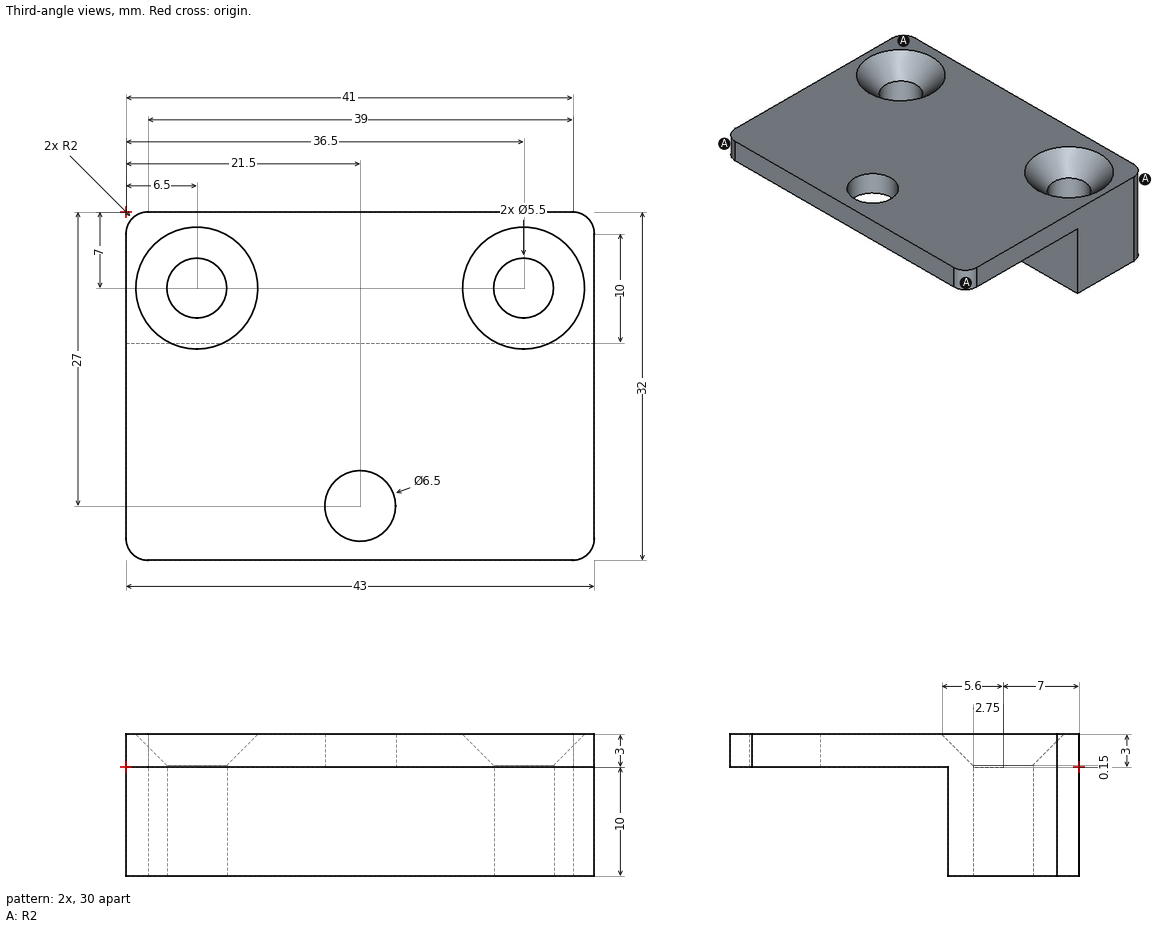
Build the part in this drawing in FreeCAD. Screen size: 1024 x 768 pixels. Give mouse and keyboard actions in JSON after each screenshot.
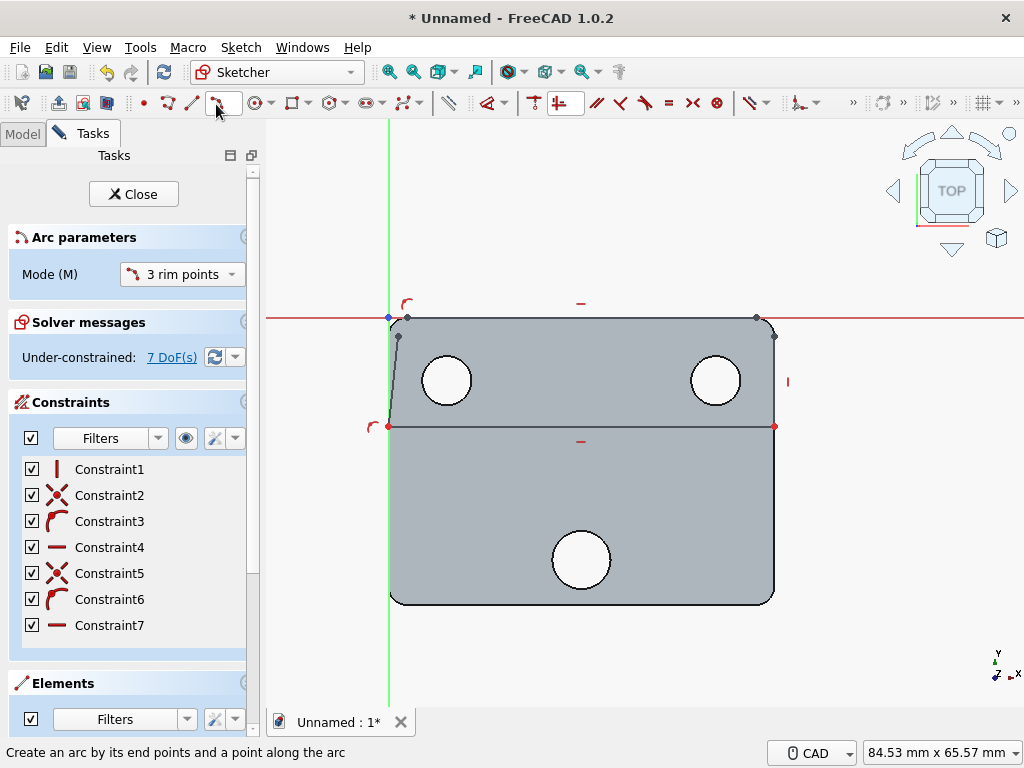
{"action": "left_click", "coordinate": [398, 337]}
{"action": "left_click", "coordinate": [407, 318]}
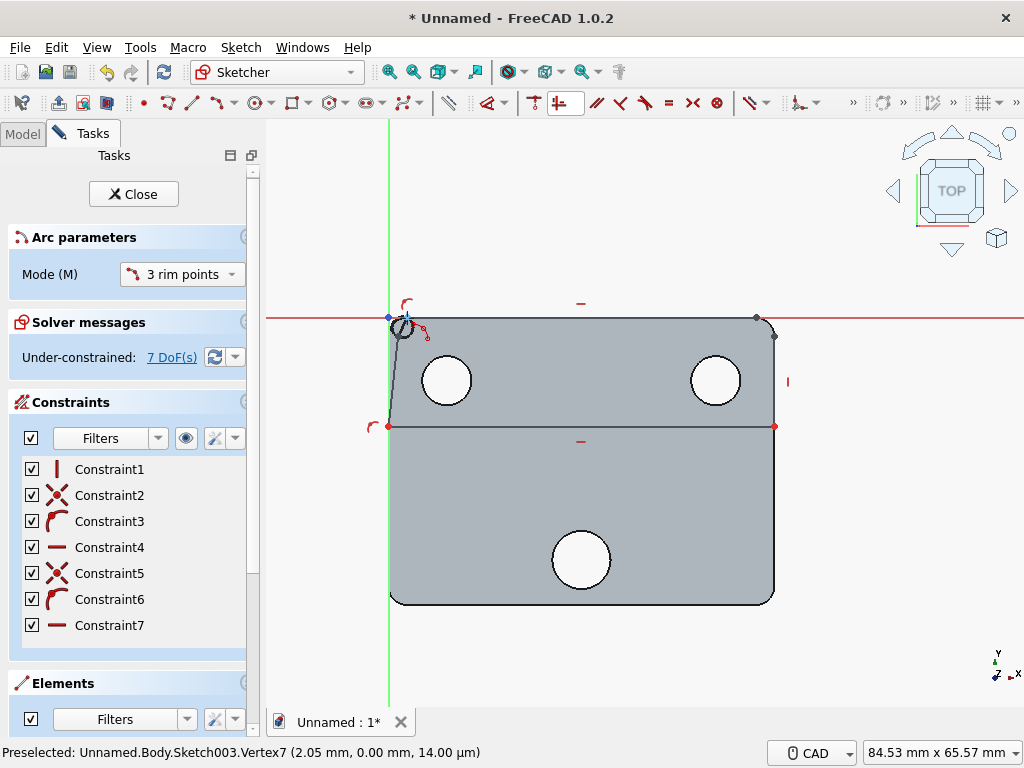
{"action": "scroll", "coordinate": [394, 323], "scroll_direction": "up", "scroll_amount": 6}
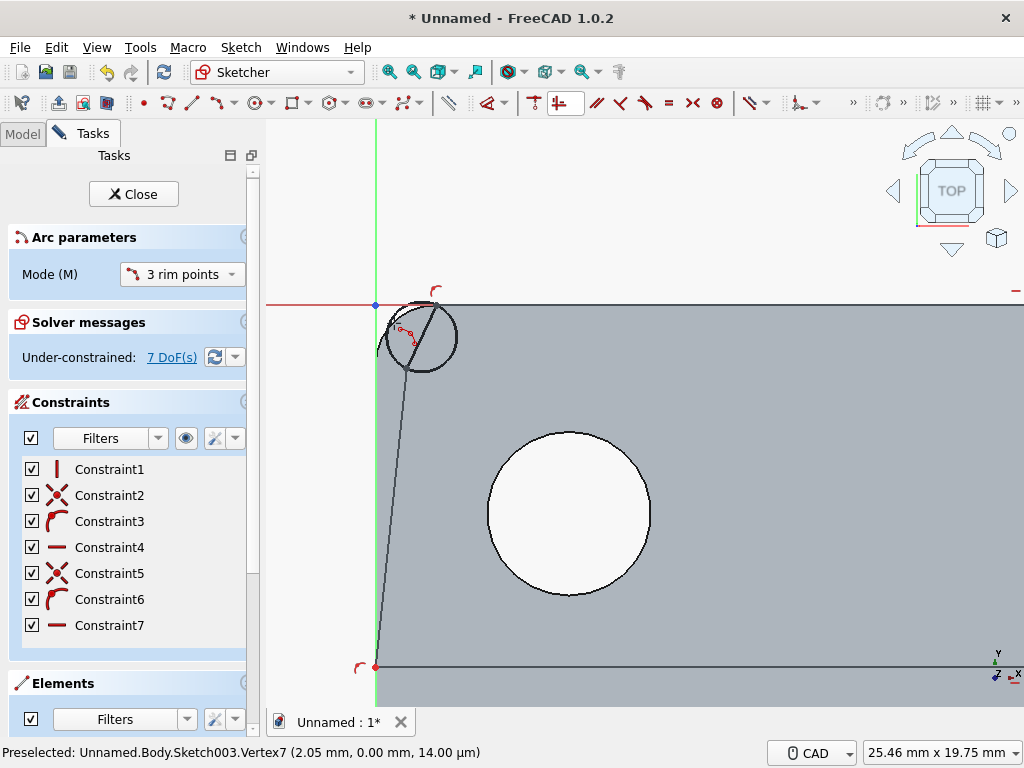
{"action": "left_click", "coordinate": [393, 323]}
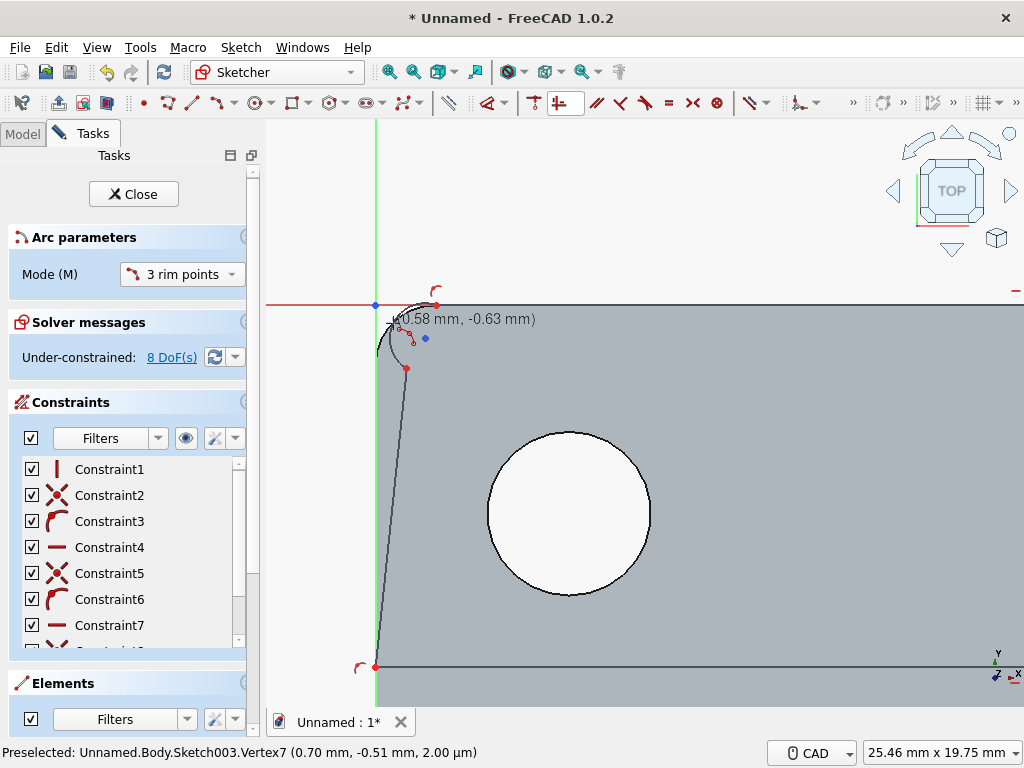
{"action": "scroll", "coordinate": [387, 382], "scroll_direction": "down", "scroll_amount": 6}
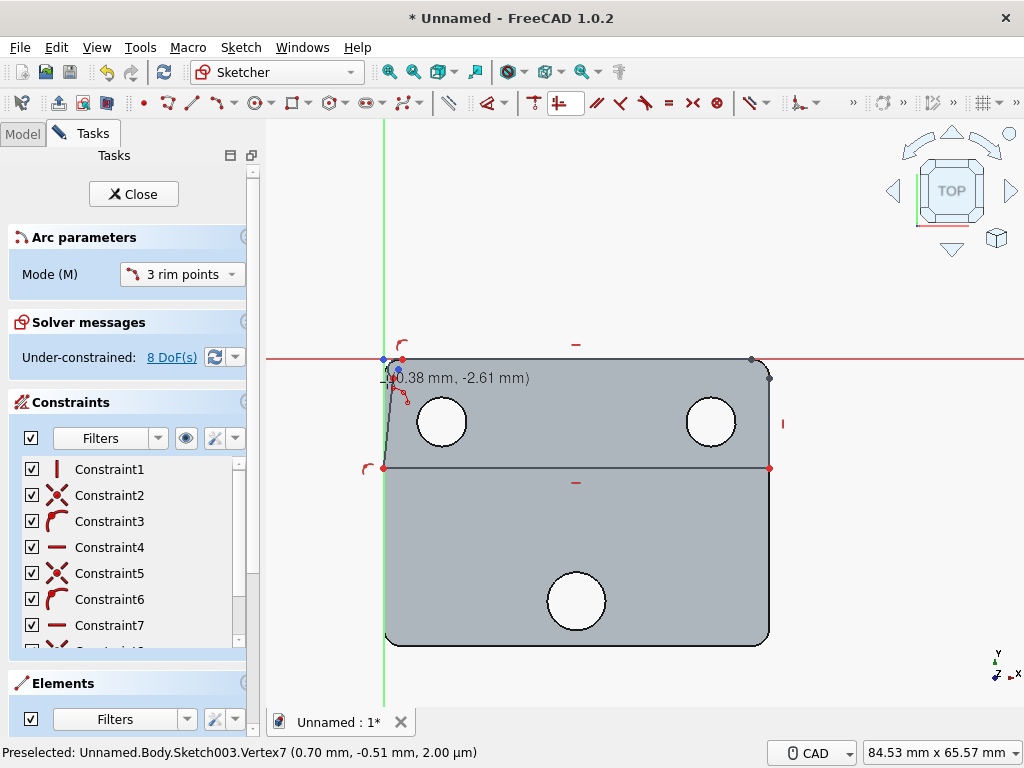
{"action": "left_click", "coordinate": [751, 368]}
{"action": "left_click", "coordinate": [769, 378]}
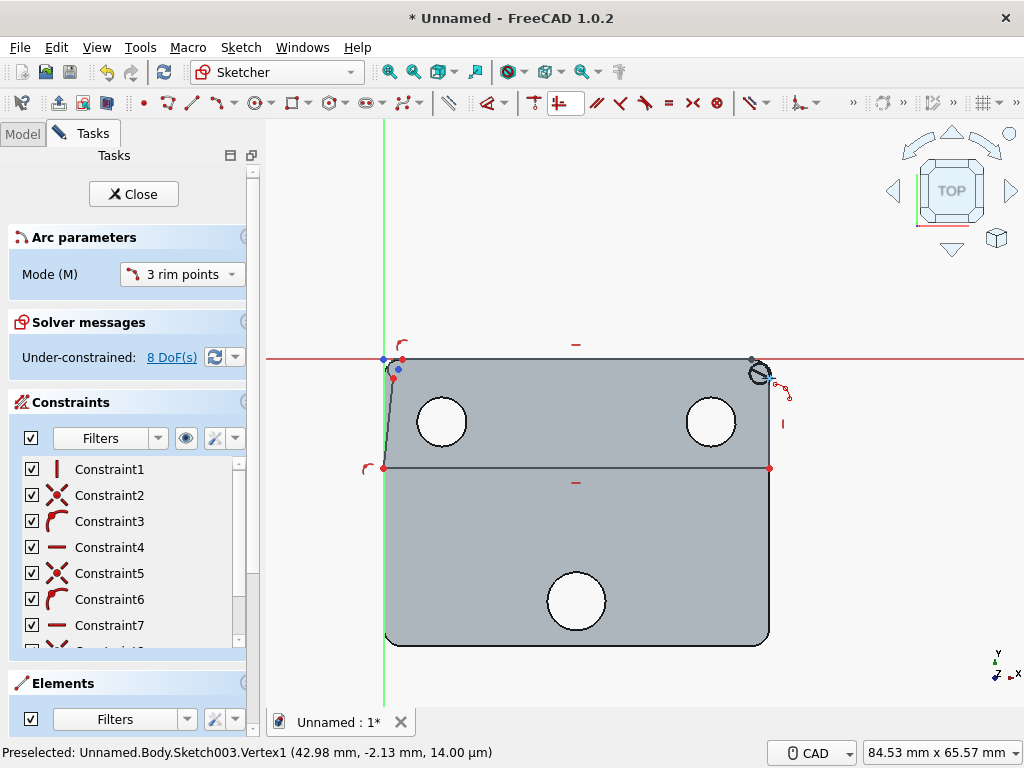
{"action": "scroll", "coordinate": [764, 364], "scroll_direction": "up", "scroll_amount": 6}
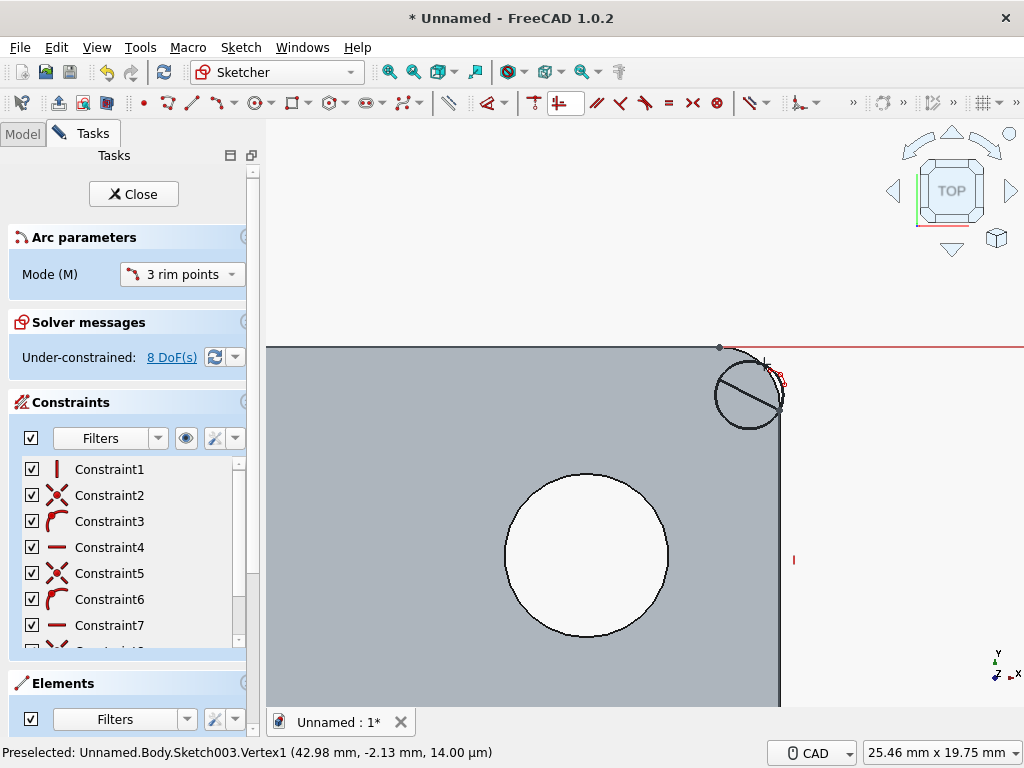
{"action": "left_click", "coordinate": [763, 365]}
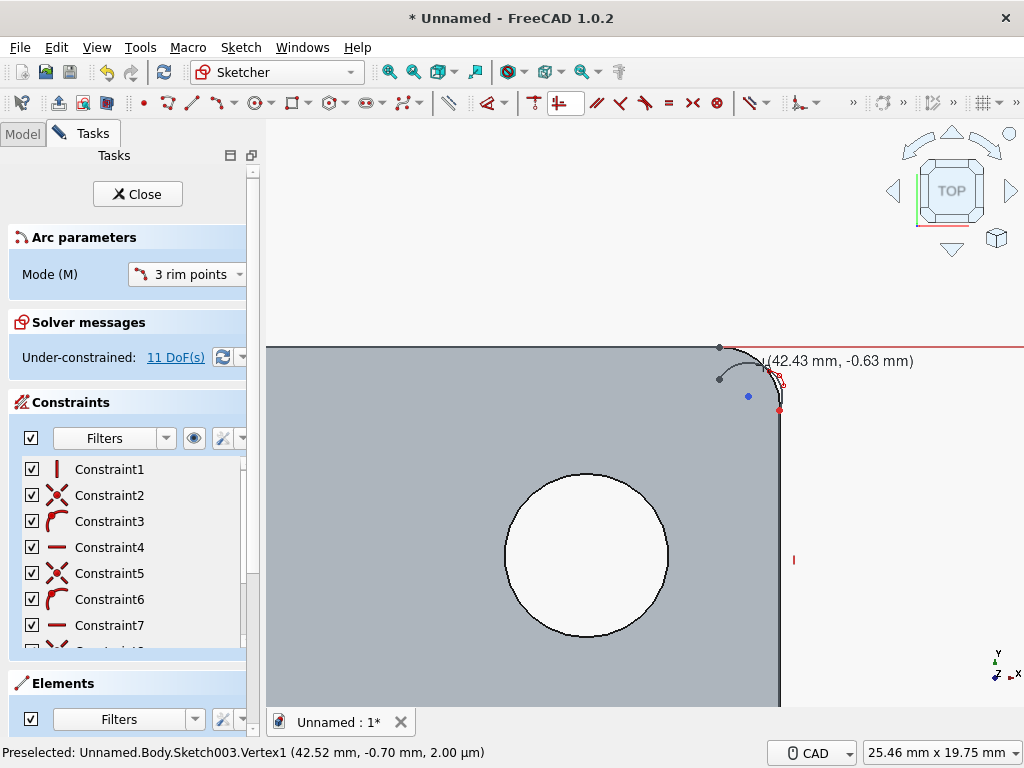
{"action": "left_click", "coordinate": [256, 104]}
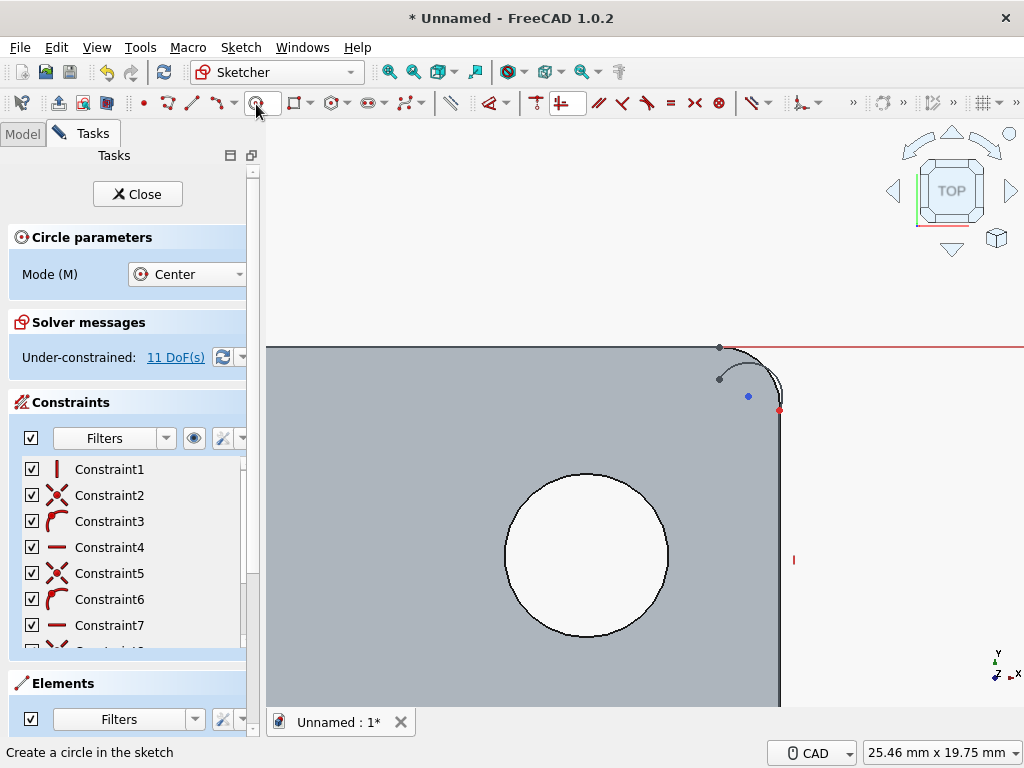
{"action": "left_click", "coordinate": [586, 556]}
{"action": "mouse_move", "coordinate": [644, 498]}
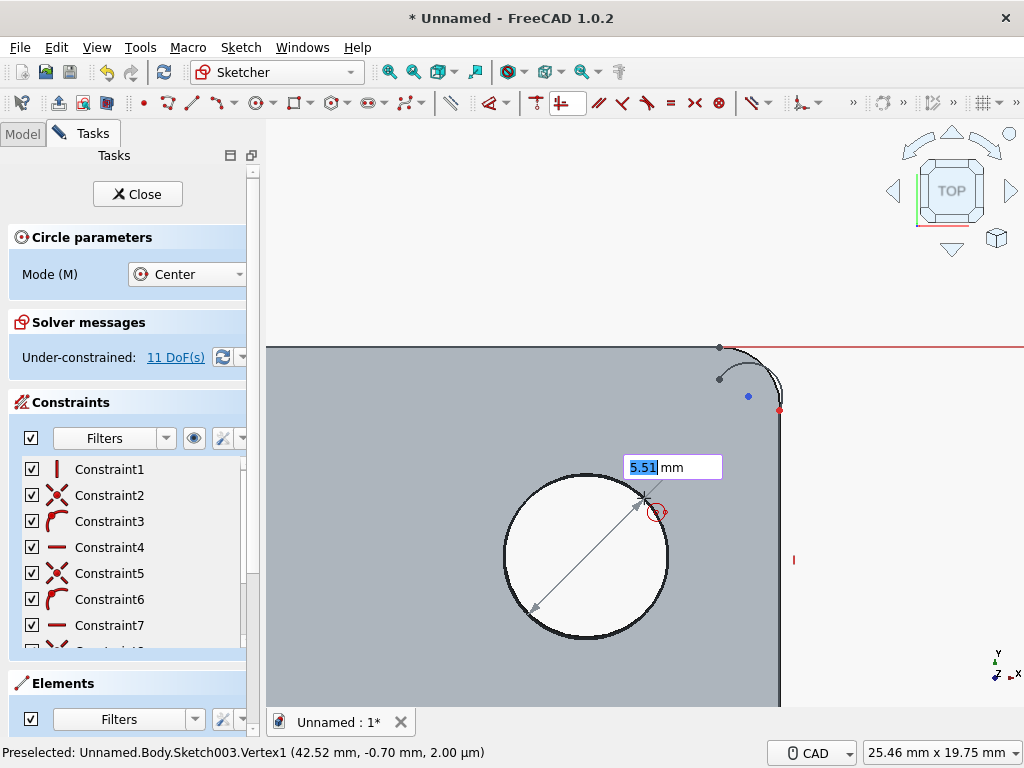
{"action": "type", "text": "5.5"}
{"action": "key", "text": "Return"}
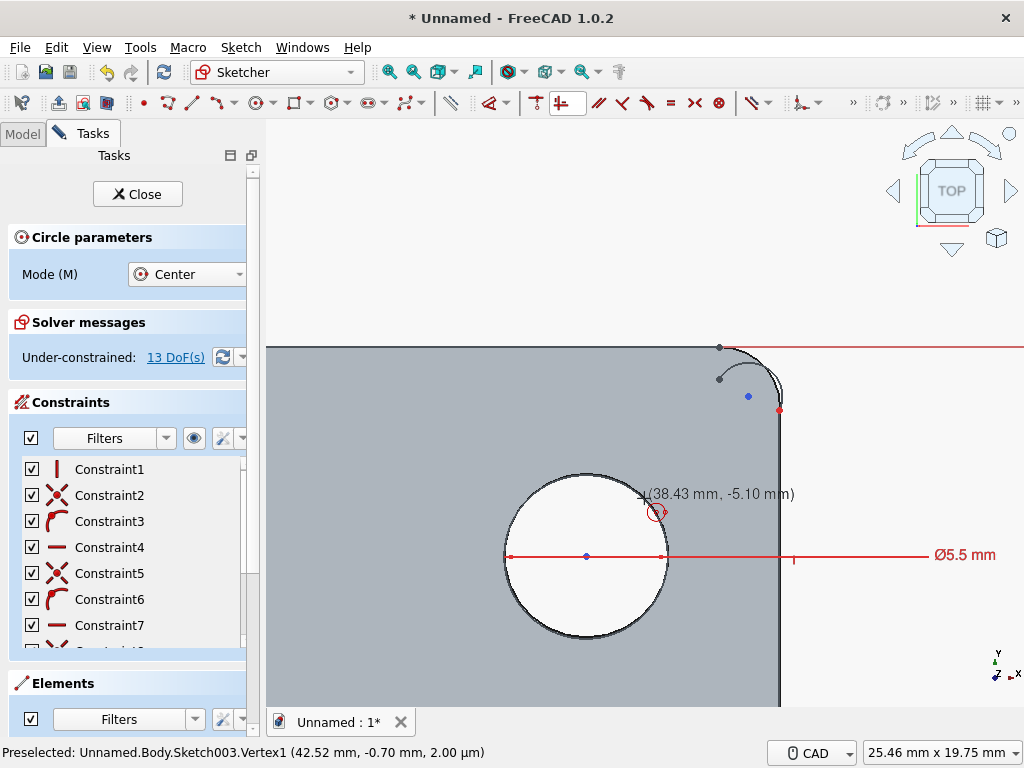
{"action": "scroll", "coordinate": [765, 364], "scroll_direction": "down", "scroll_amount": 6}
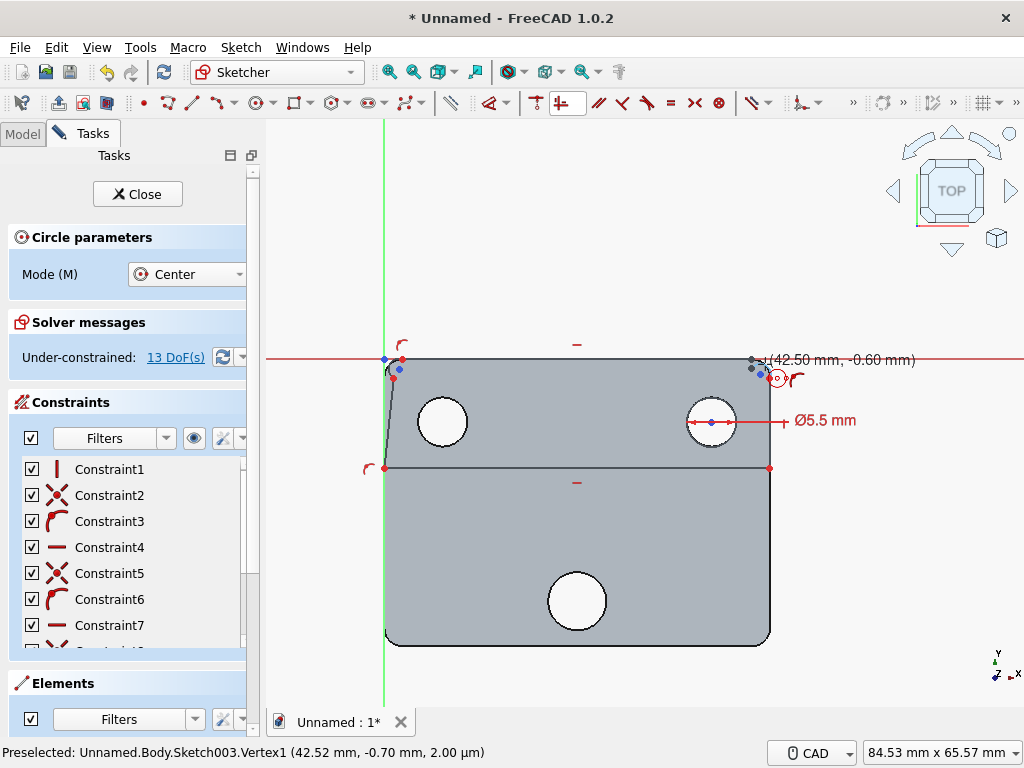
{"action": "left_click", "coordinate": [443, 422]}
{"action": "mouse_move", "coordinate": [460, 405]}